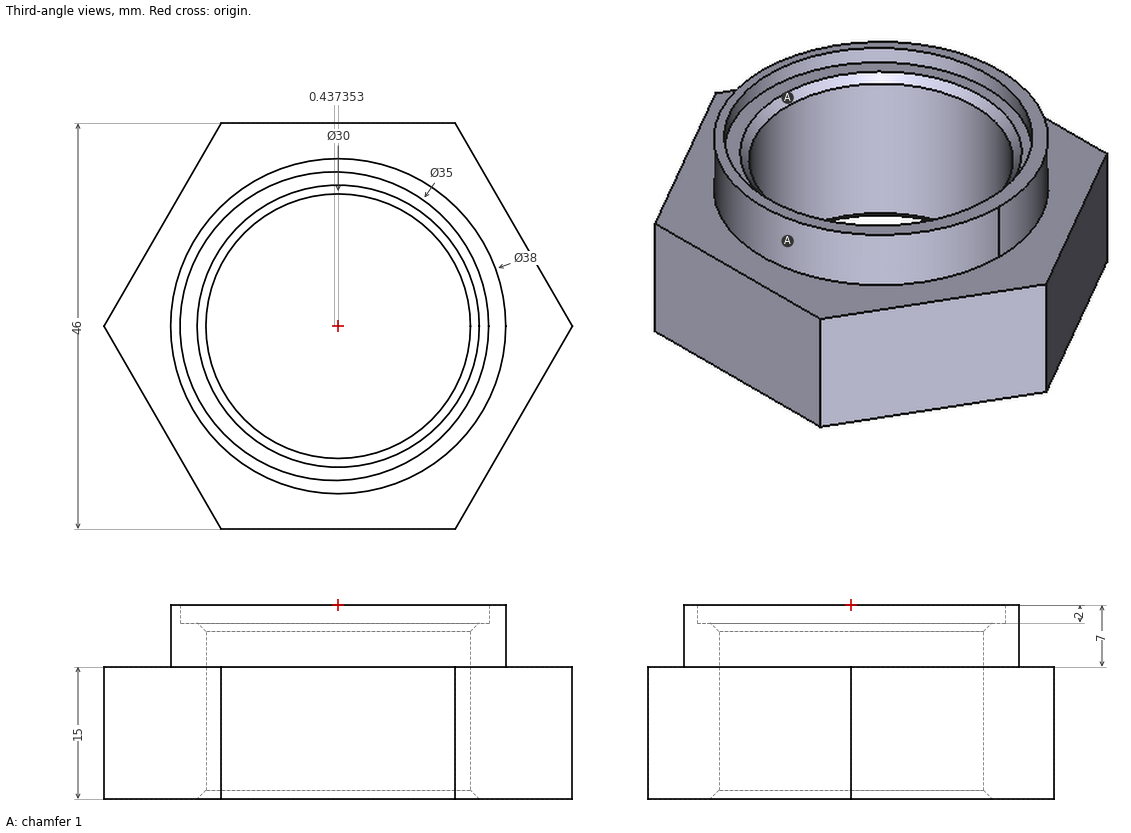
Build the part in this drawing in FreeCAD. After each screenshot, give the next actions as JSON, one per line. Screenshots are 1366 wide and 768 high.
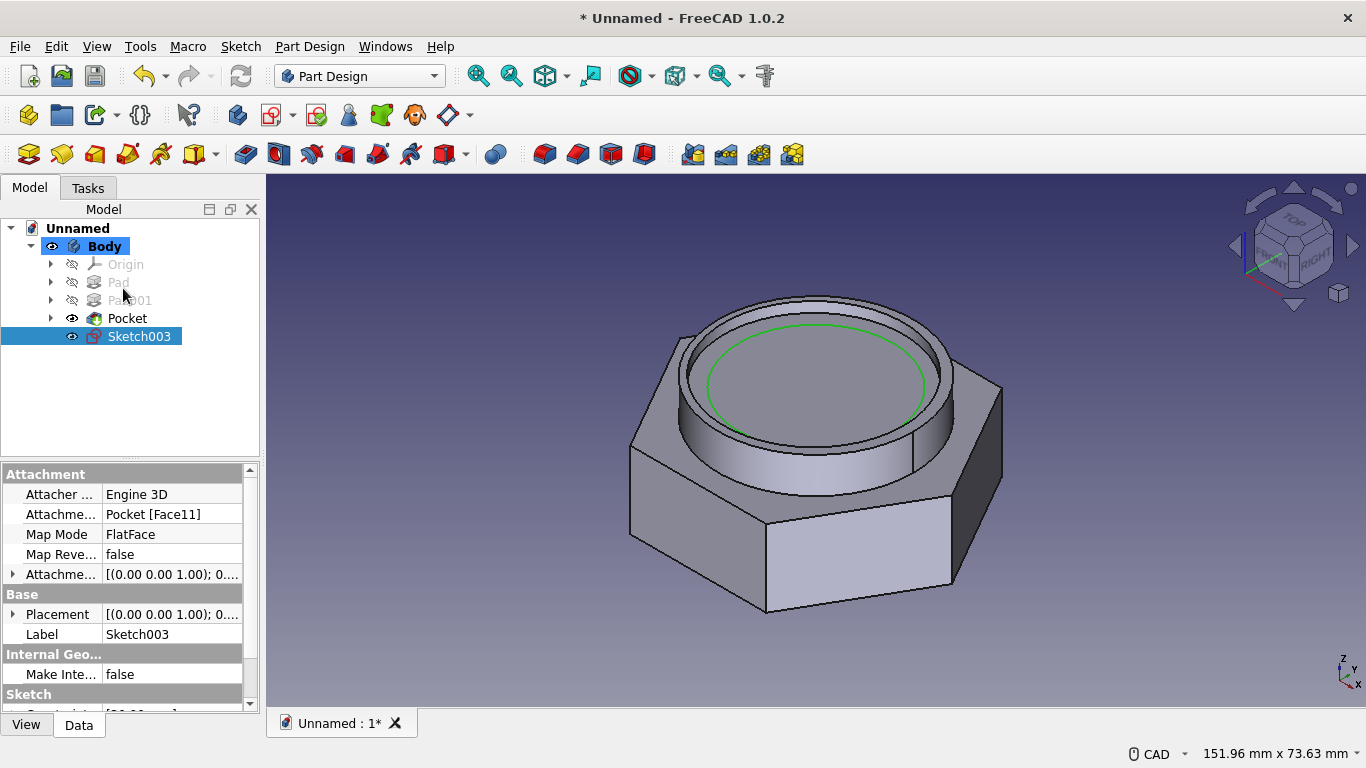
{"action": "left_click", "coordinate": [246, 154]}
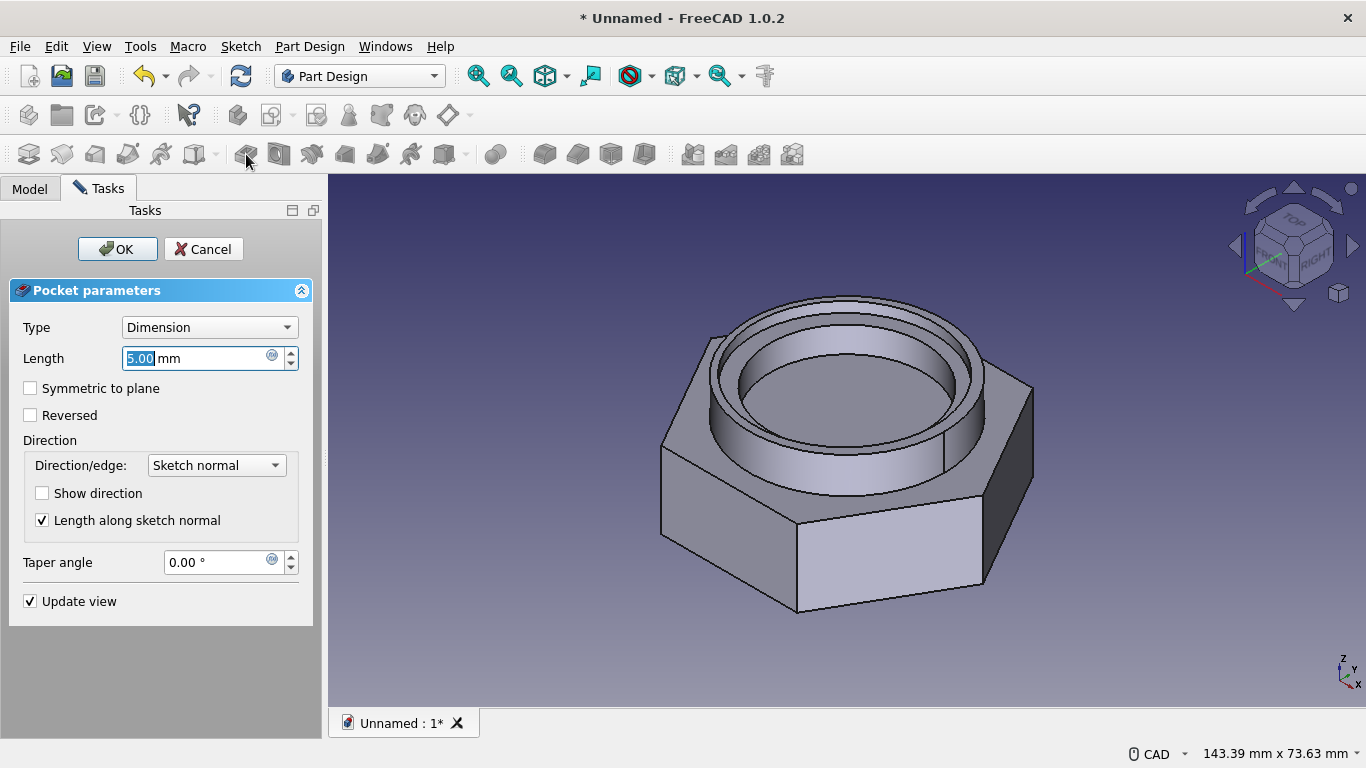
{"action": "left_click", "coordinate": [210, 328]}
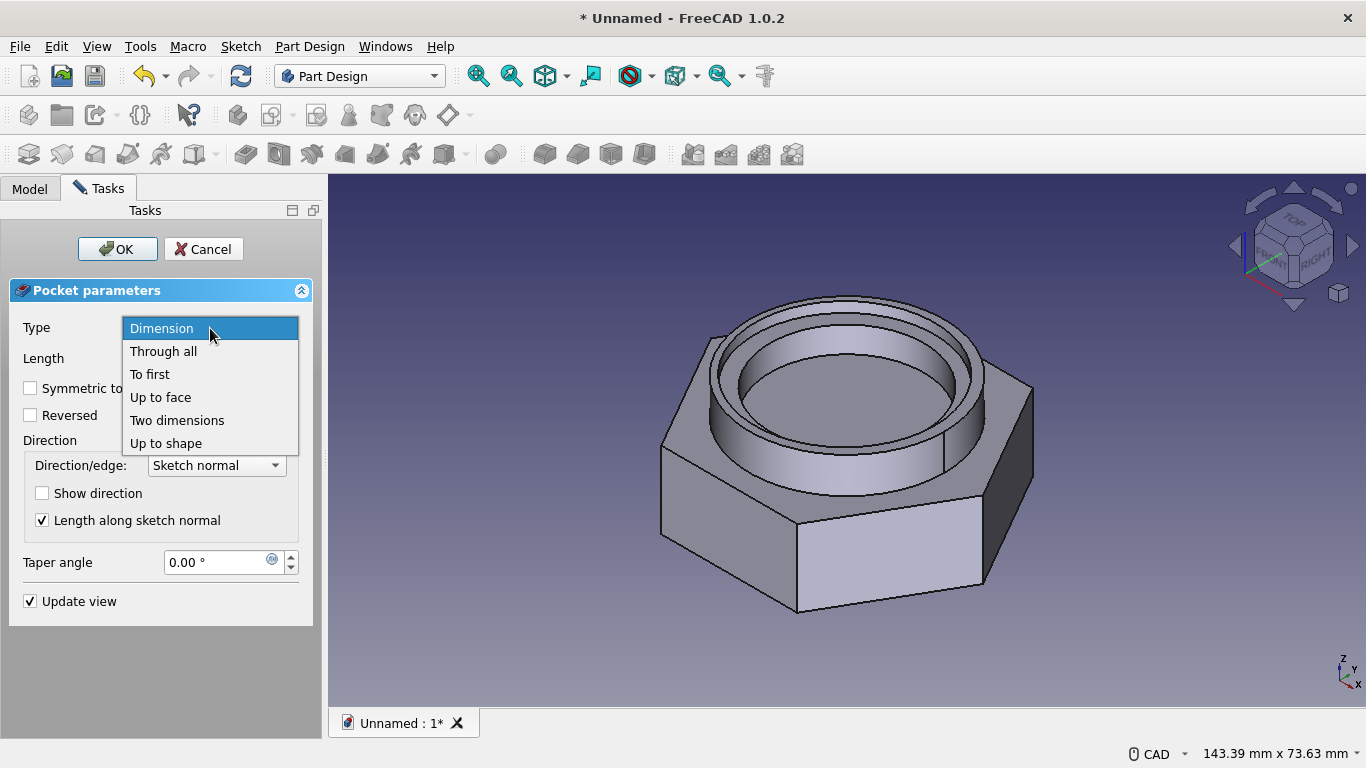
{"action": "left_click", "coordinate": [208, 352]}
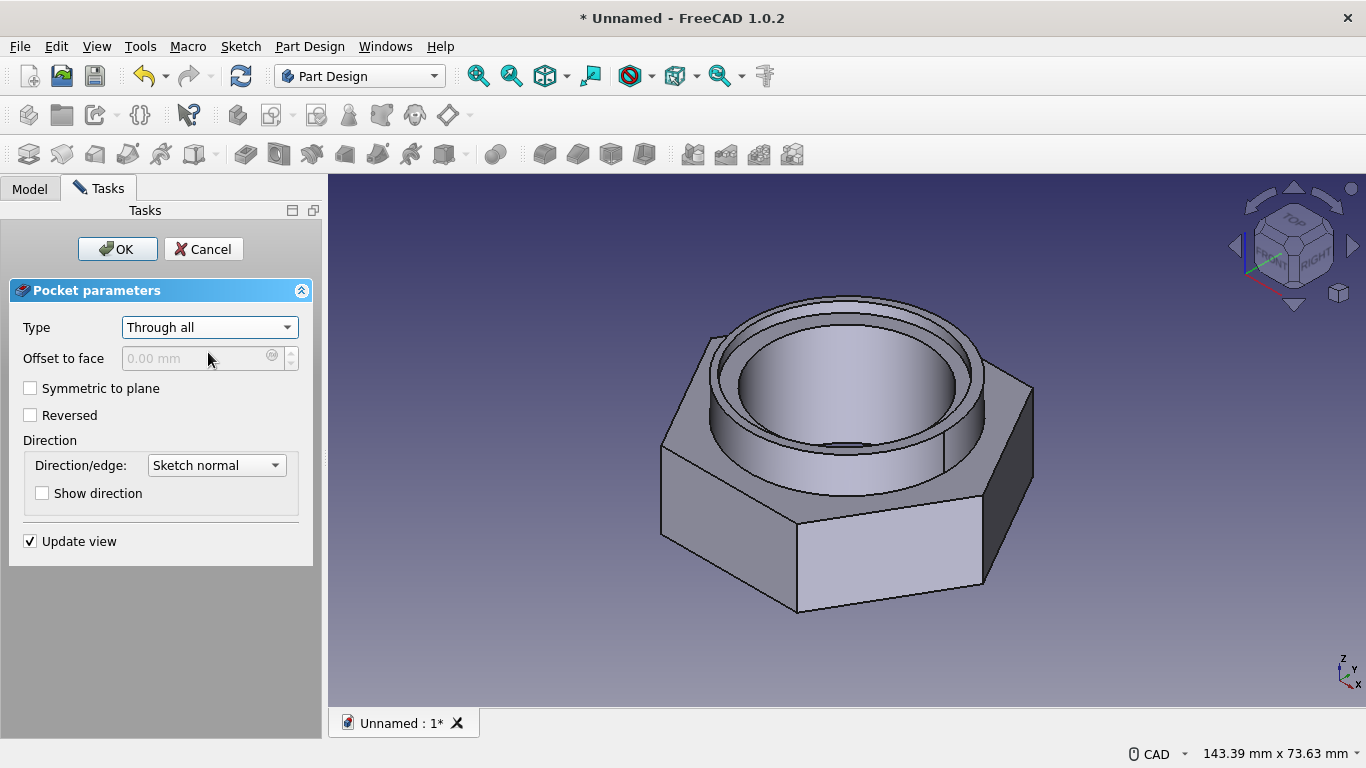
{"action": "left_click", "coordinate": [118, 249]}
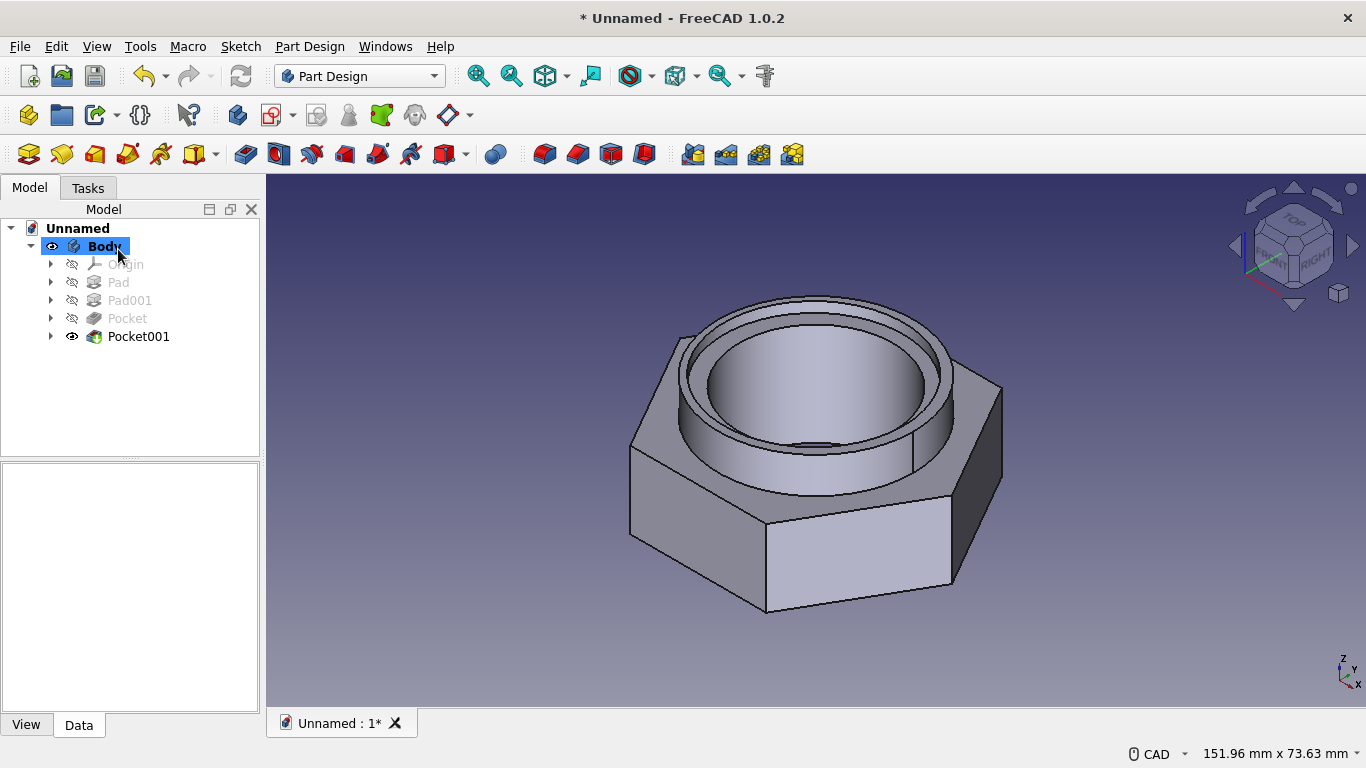
{"action": "left_click", "coordinate": [739, 342]}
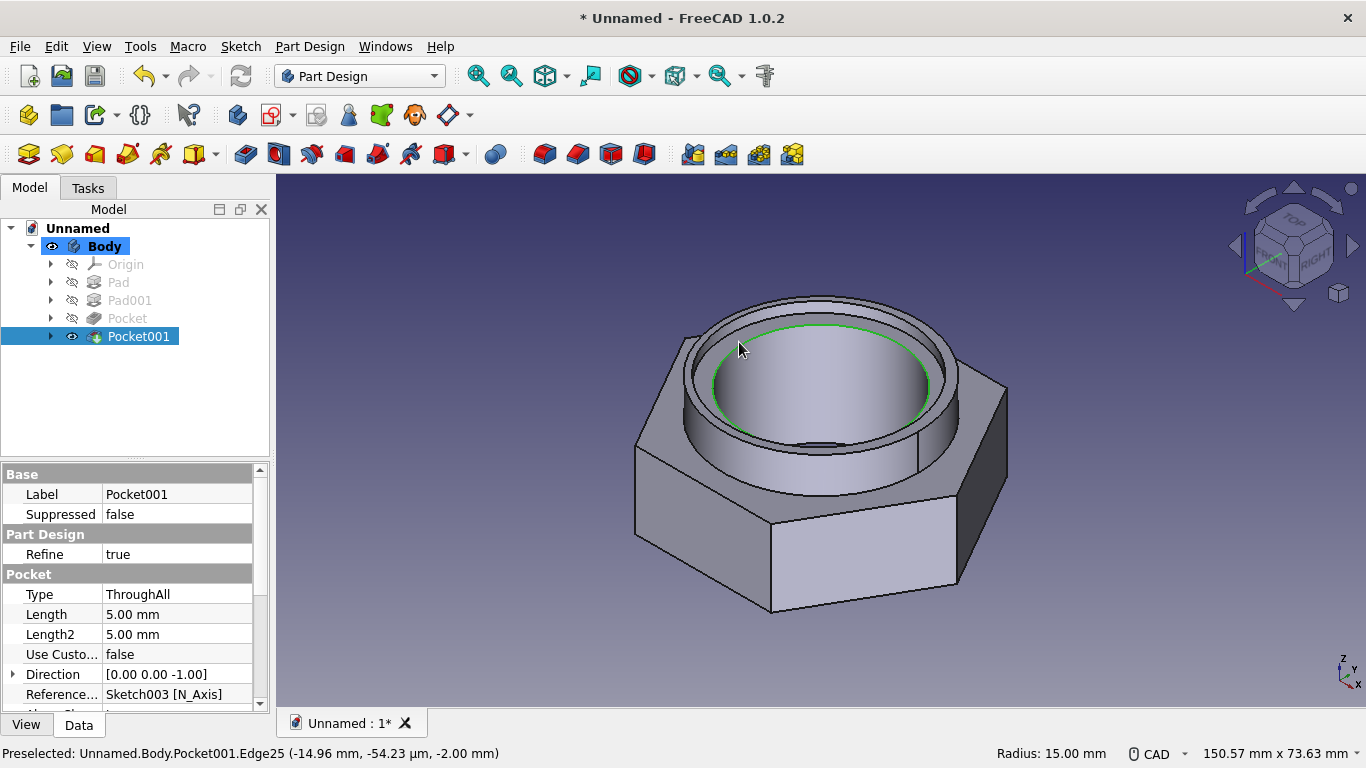
{"action": "key", "text": "2"}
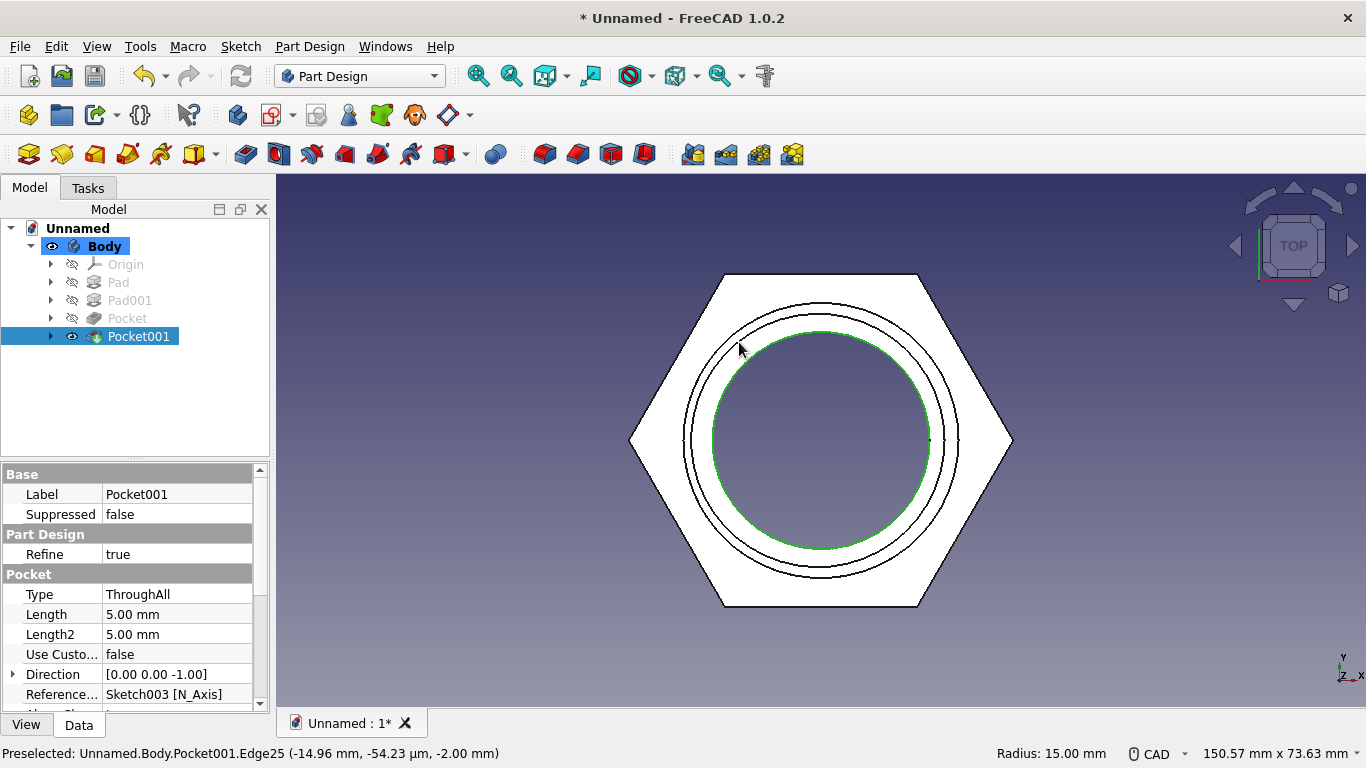
{"action": "key", "text": "0"}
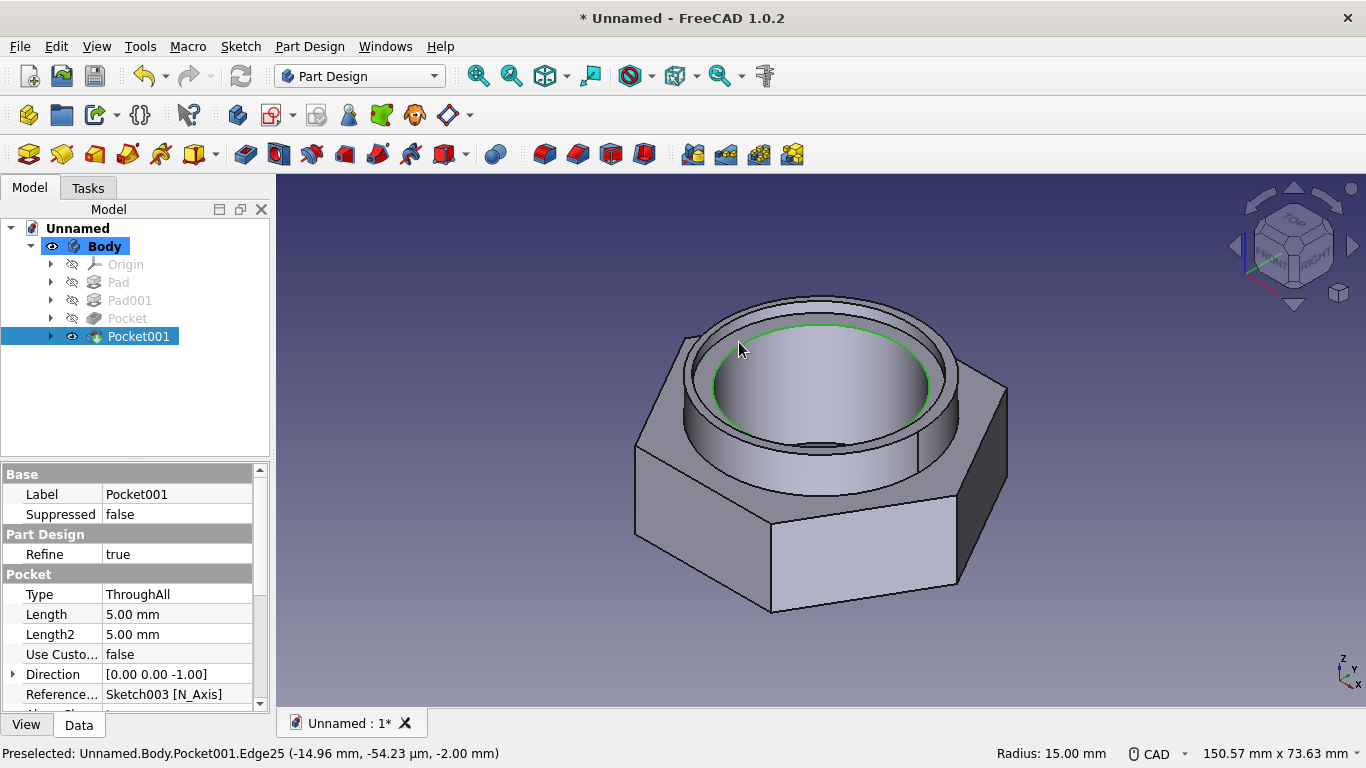
{"action": "key", "text": "1"}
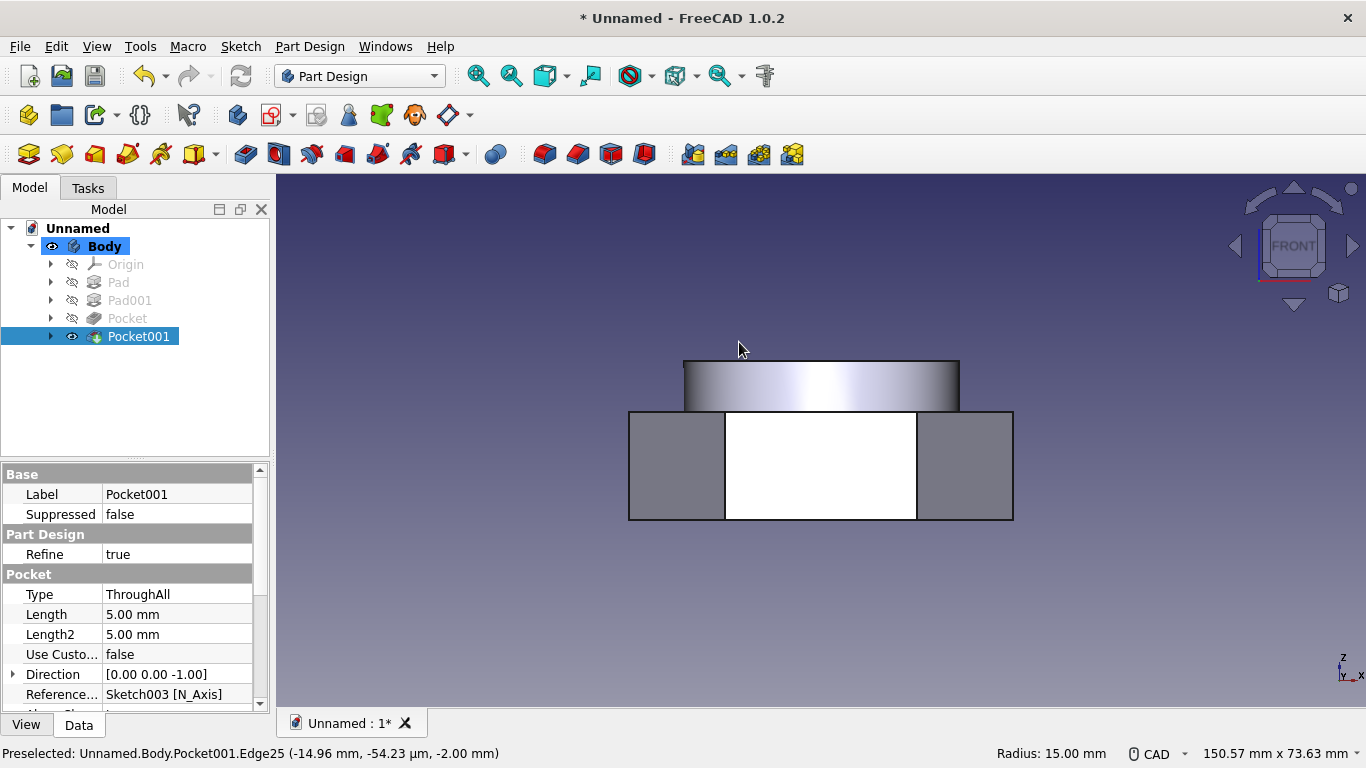
{"action": "left_click", "coordinate": [479, 76]}